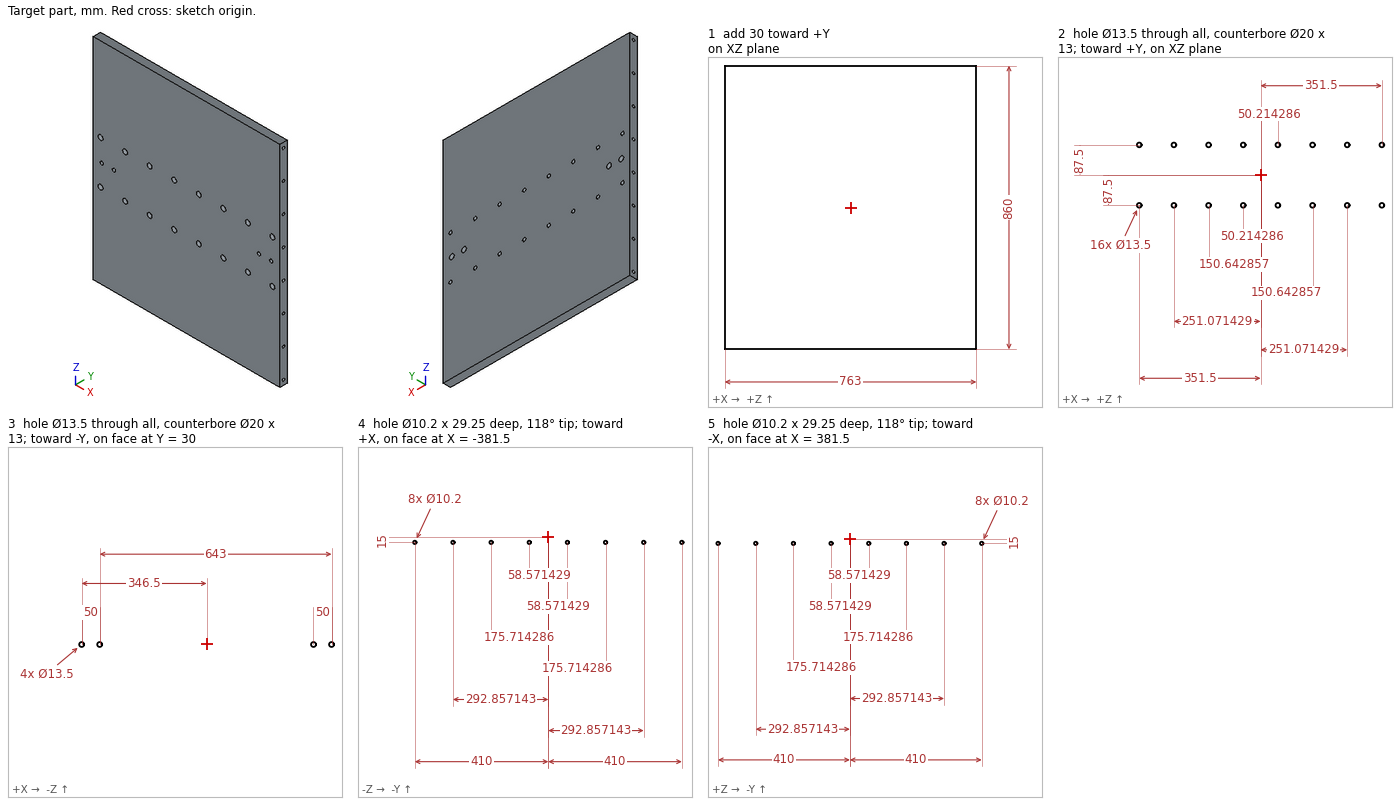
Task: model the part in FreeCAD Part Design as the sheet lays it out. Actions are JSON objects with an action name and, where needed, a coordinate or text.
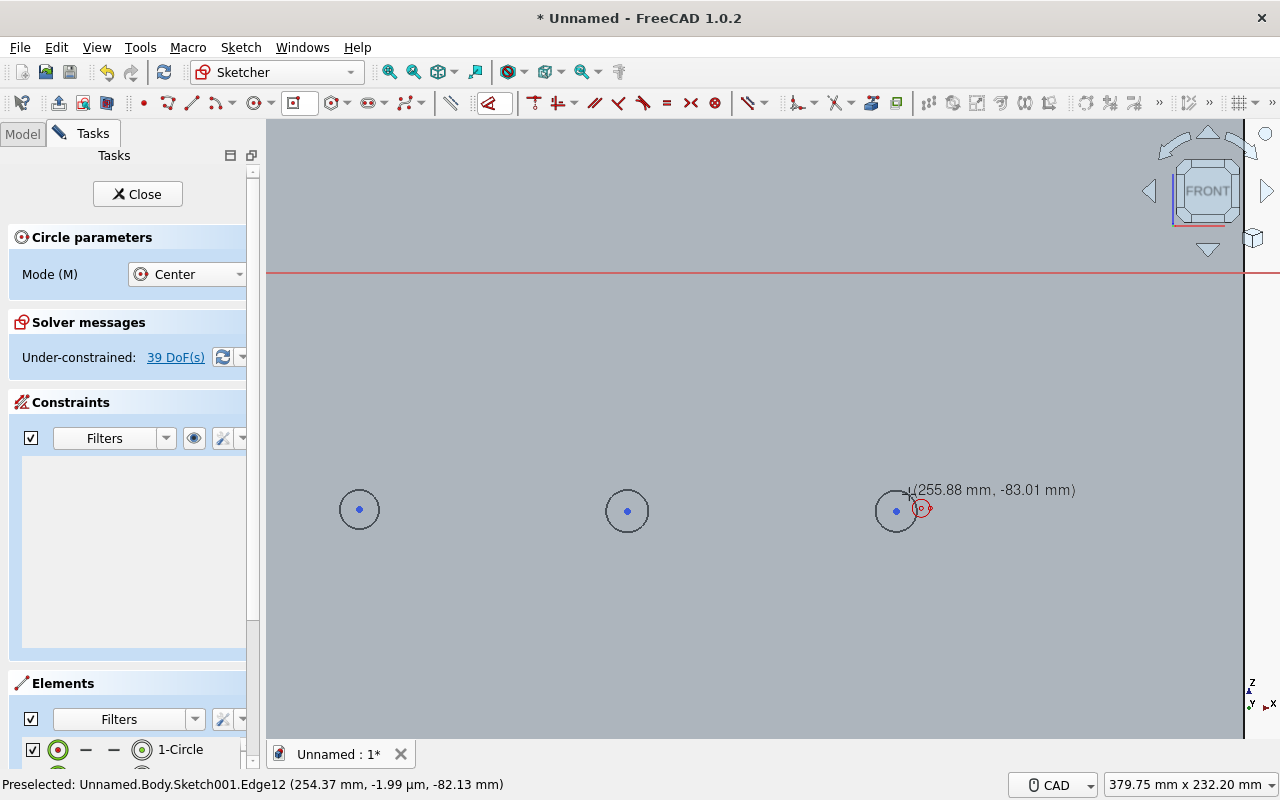
{"action": "scroll", "coordinate": [911, 496], "scroll_direction": "down", "scroll_amount": 6}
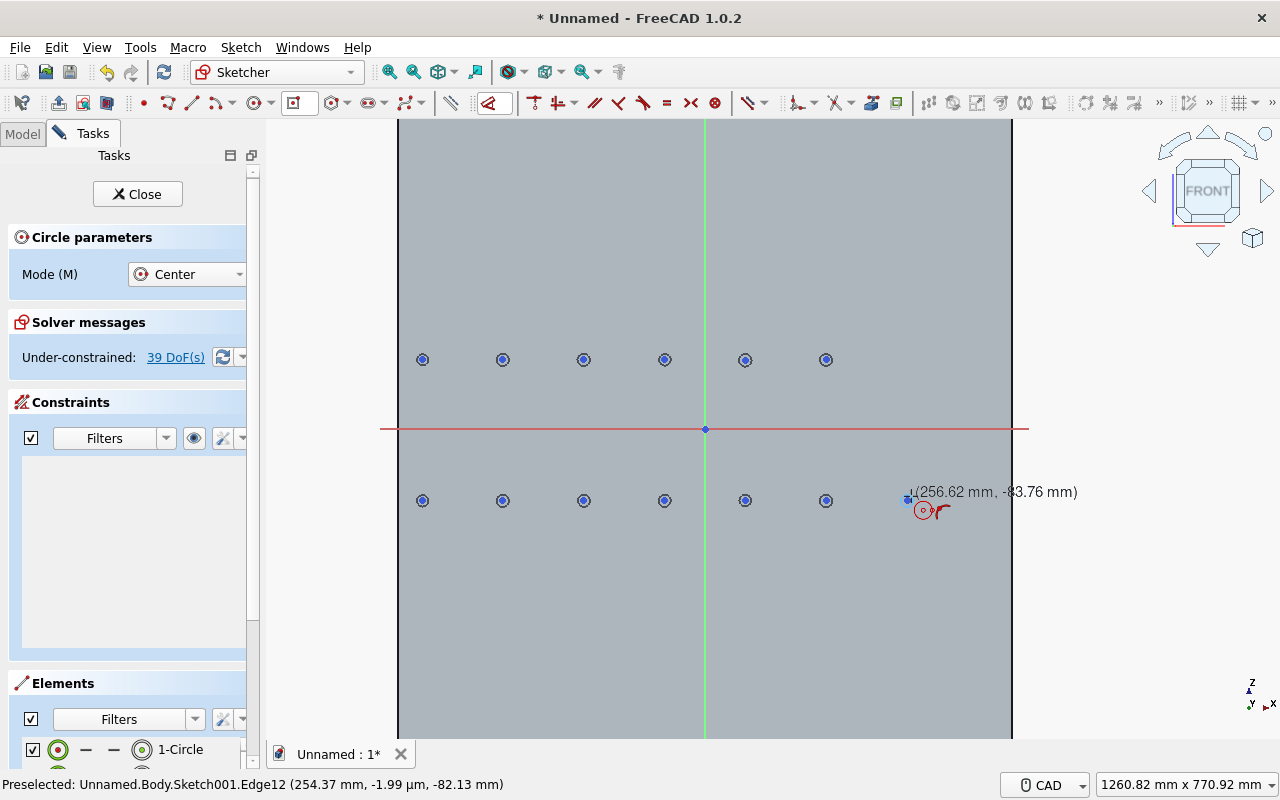
{"action": "scroll", "coordinate": [907, 359], "scroll_direction": "up", "scroll_amount": 8}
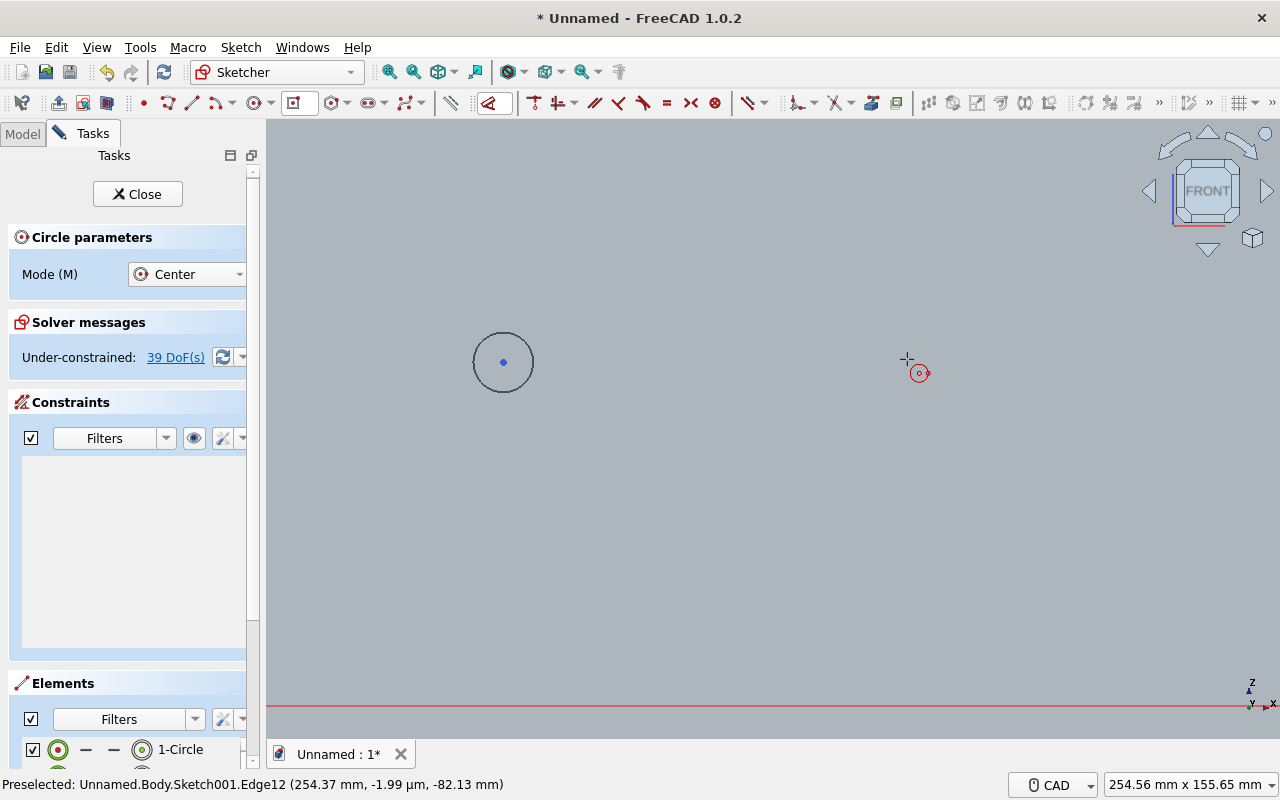
{"action": "scroll", "coordinate": [907, 359], "scroll_direction": "down", "scroll_amount": 8}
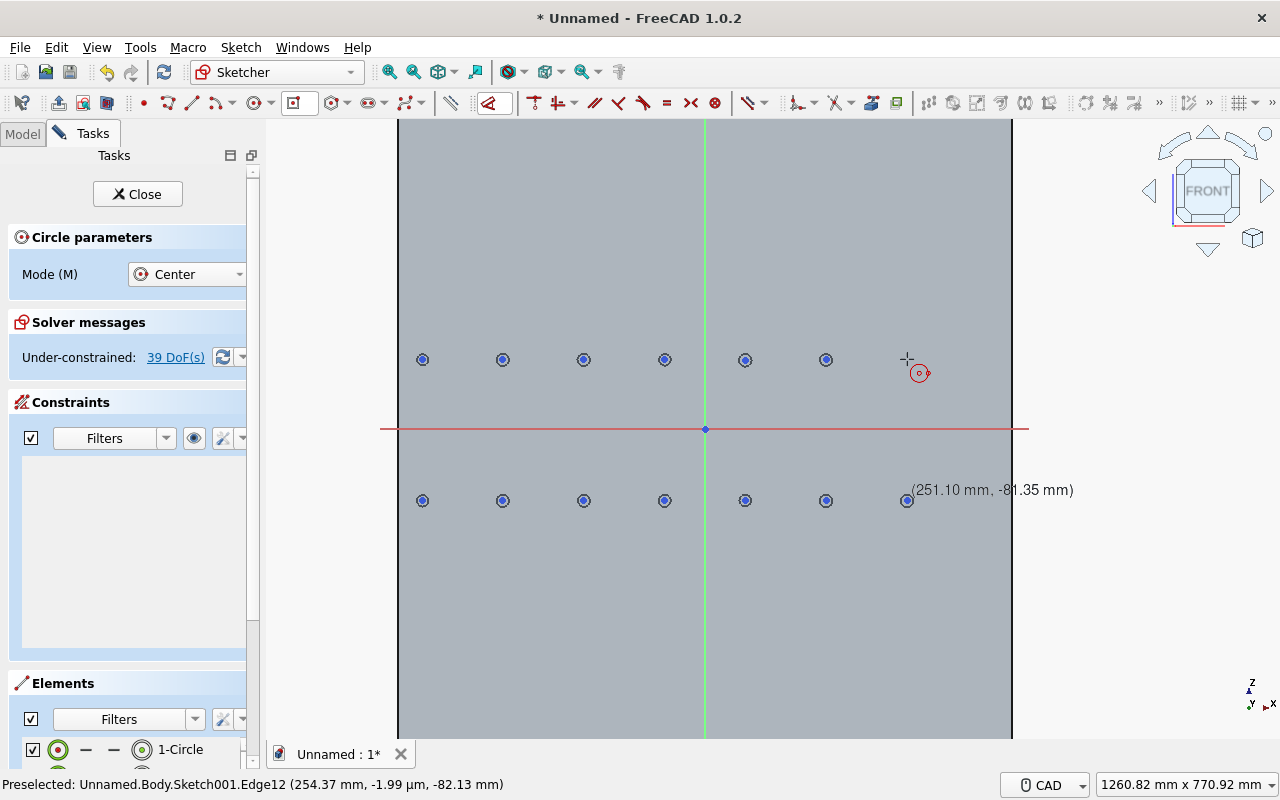
{"action": "left_click", "coordinate": [907, 359]}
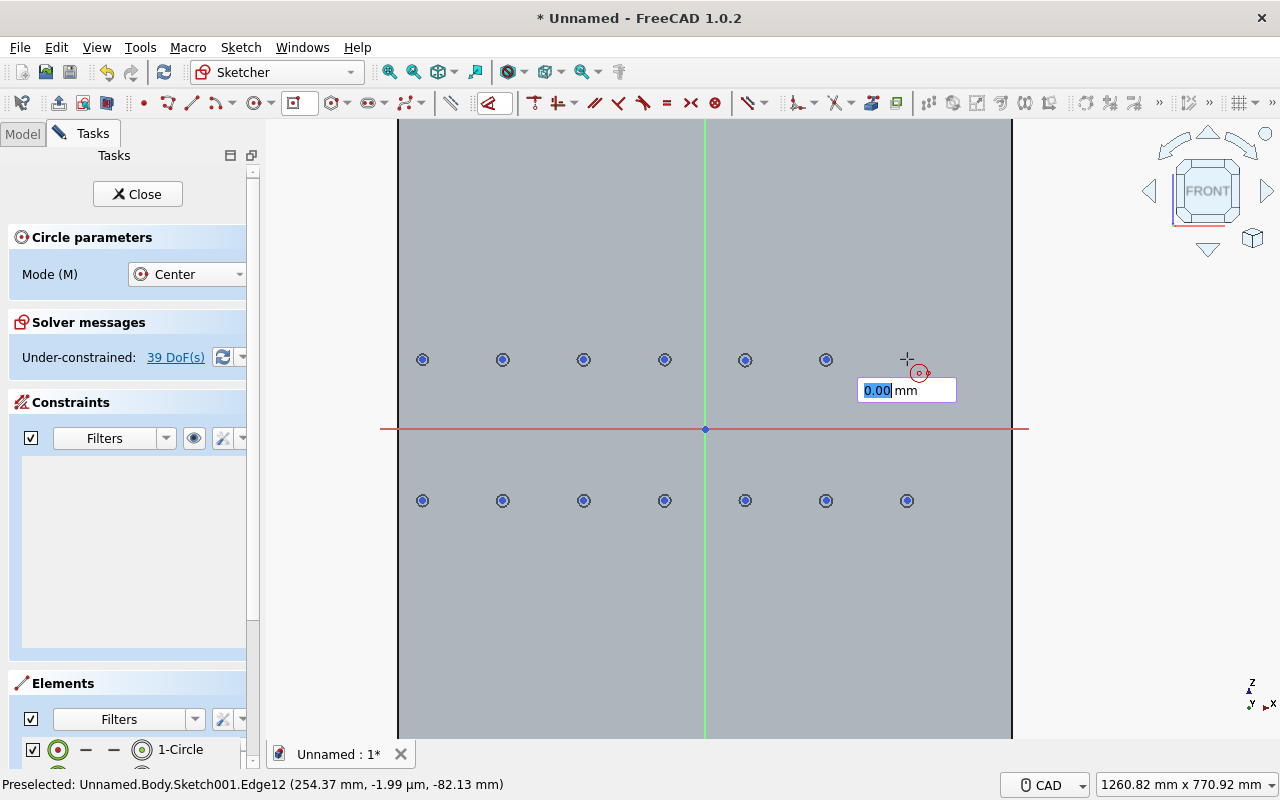
{"action": "scroll", "coordinate": [911, 355], "scroll_direction": "up", "scroll_amount": 6}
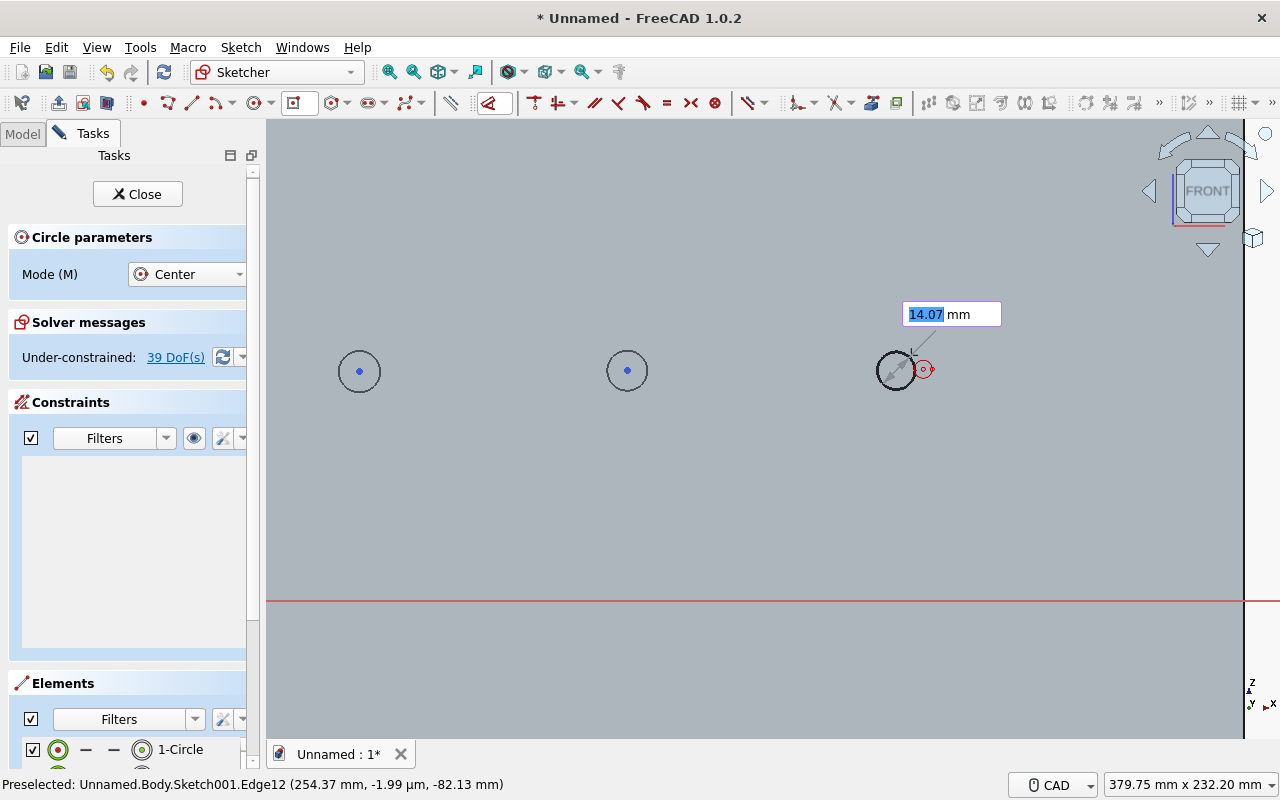
{"action": "left_click", "coordinate": [909, 355]}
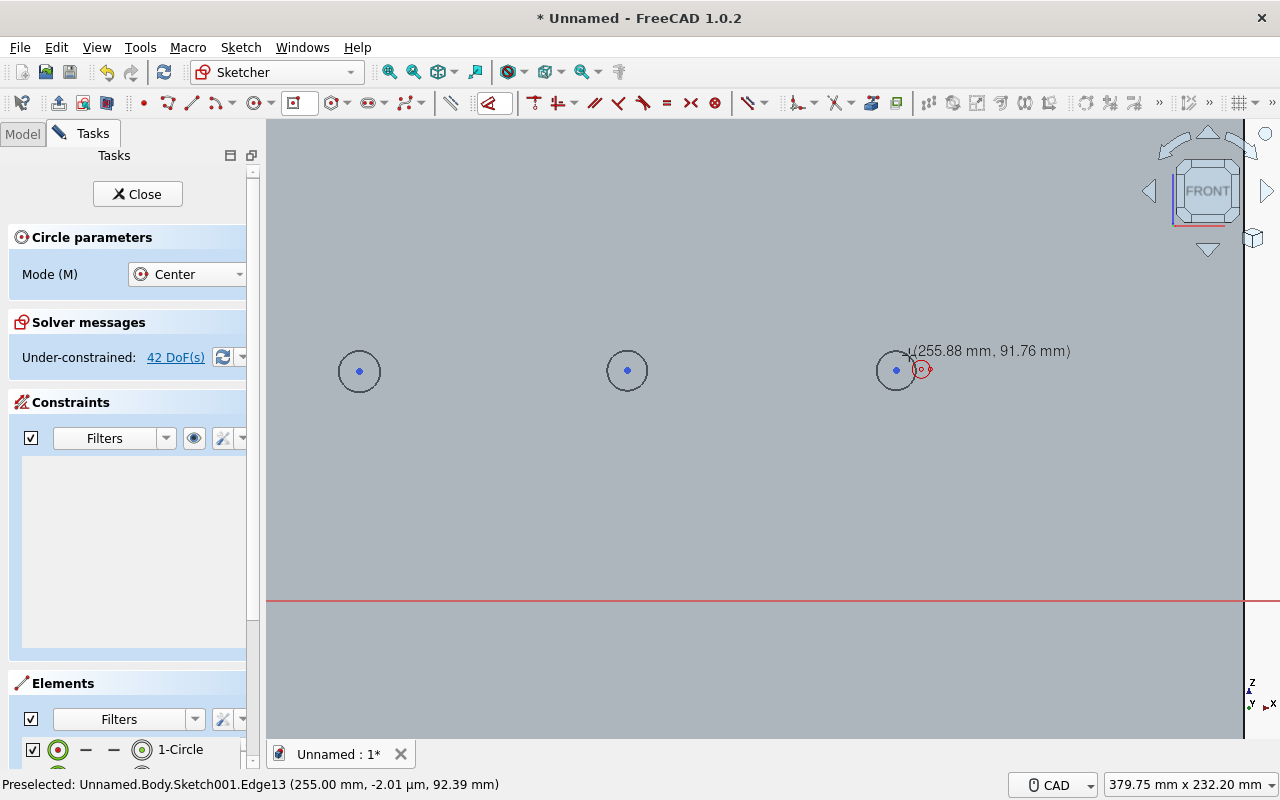
{"action": "scroll", "coordinate": [911, 355], "scroll_direction": "down", "scroll_amount": 6}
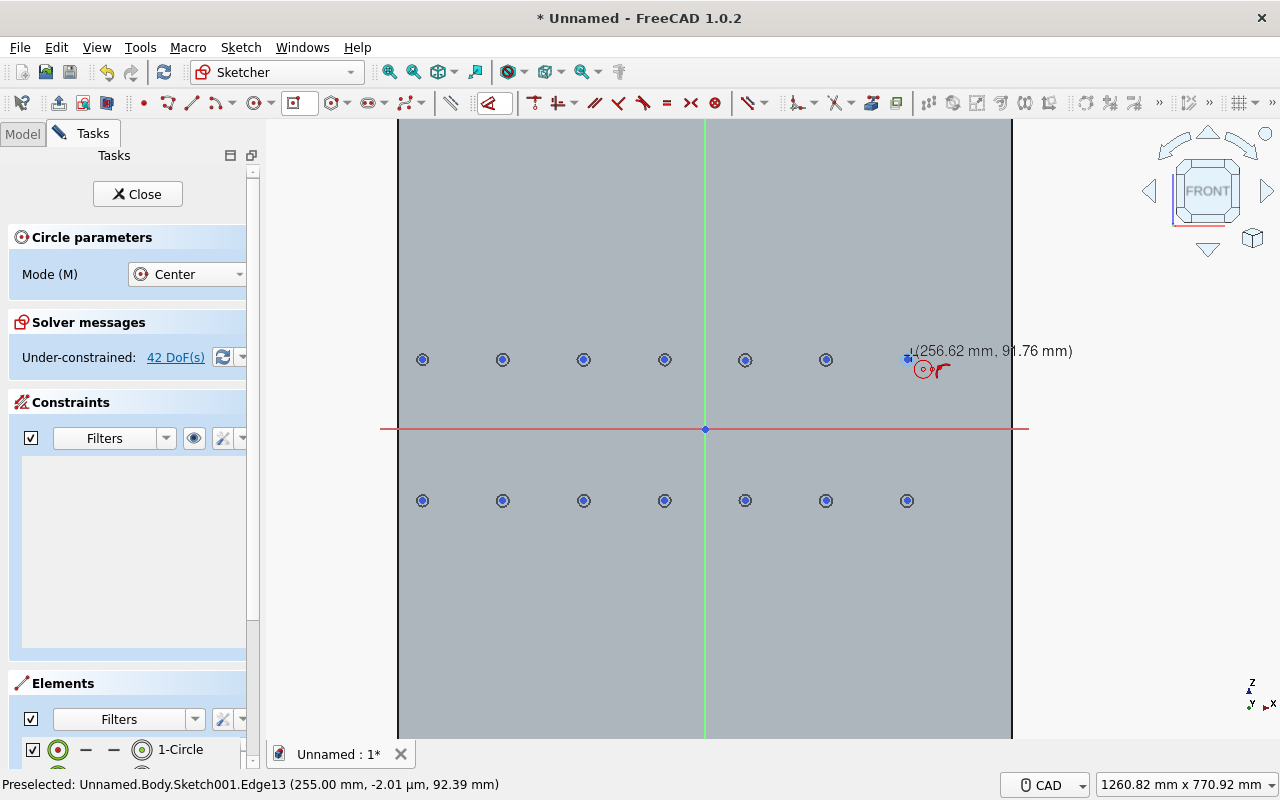
{"action": "scroll", "coordinate": [988, 359], "scroll_direction": "up", "scroll_amount": 8}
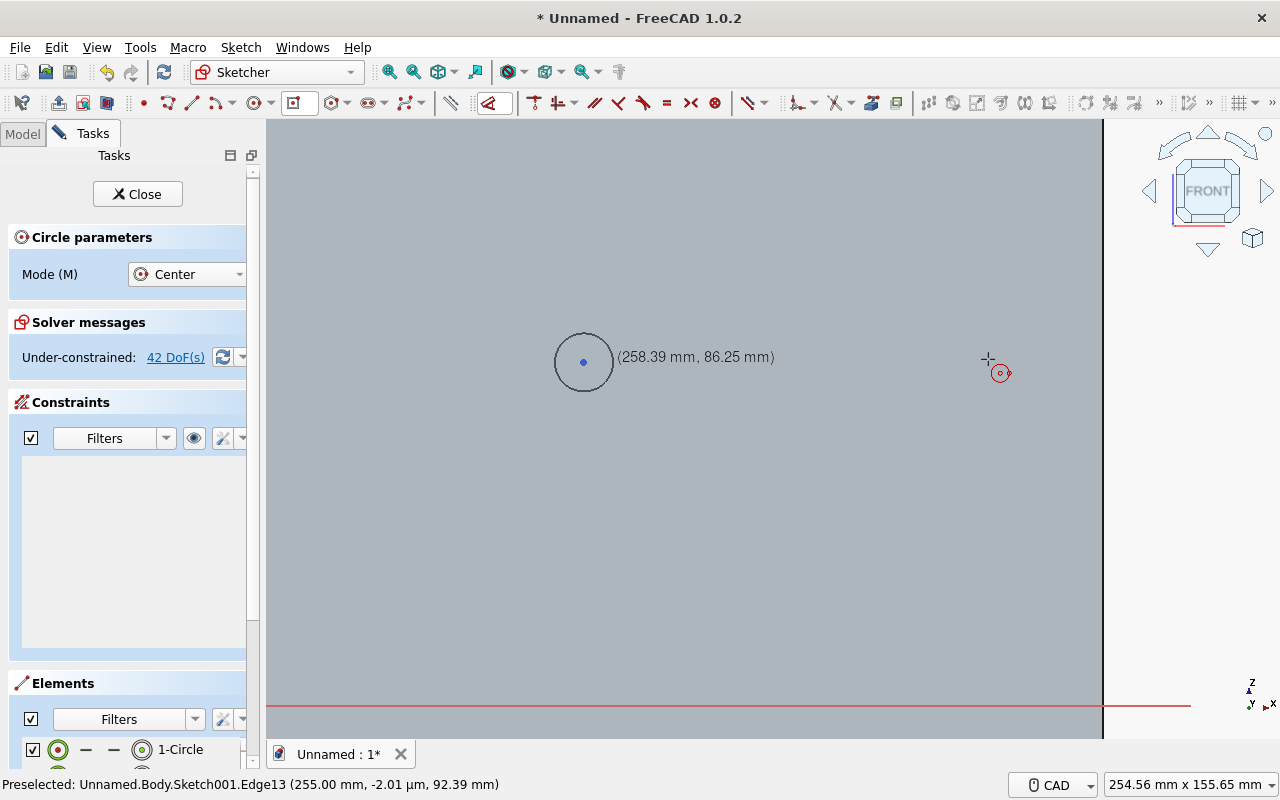
{"action": "scroll", "coordinate": [988, 359], "scroll_direction": "down", "scroll_amount": 8}